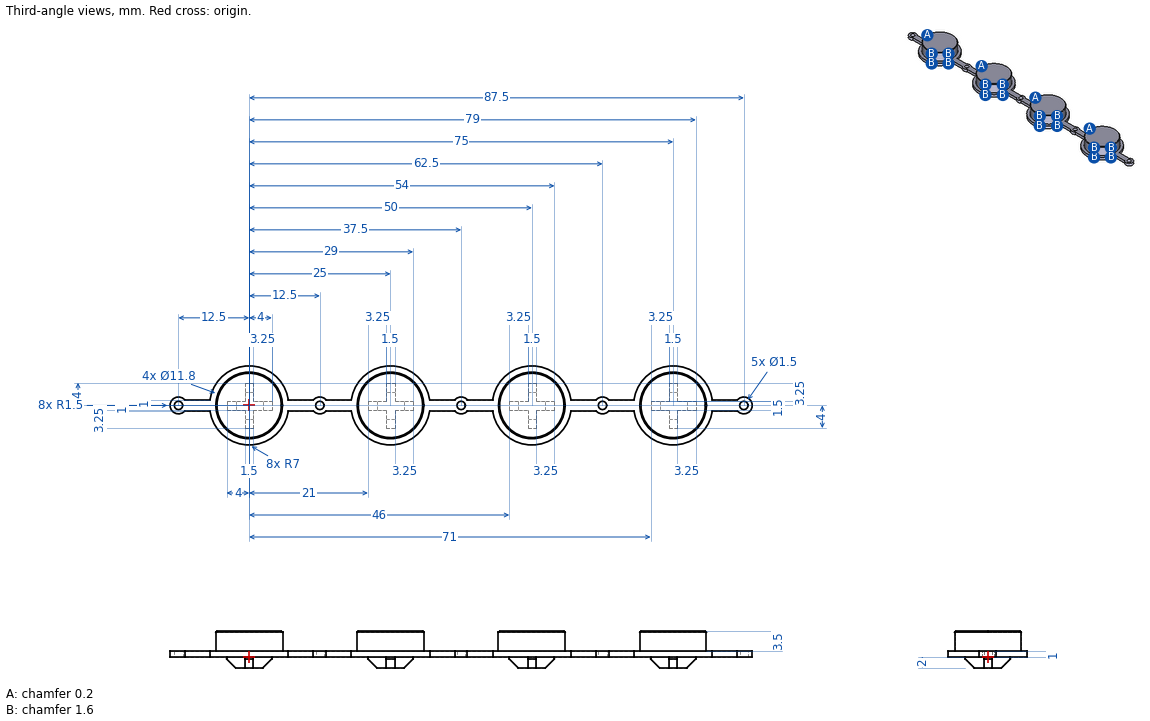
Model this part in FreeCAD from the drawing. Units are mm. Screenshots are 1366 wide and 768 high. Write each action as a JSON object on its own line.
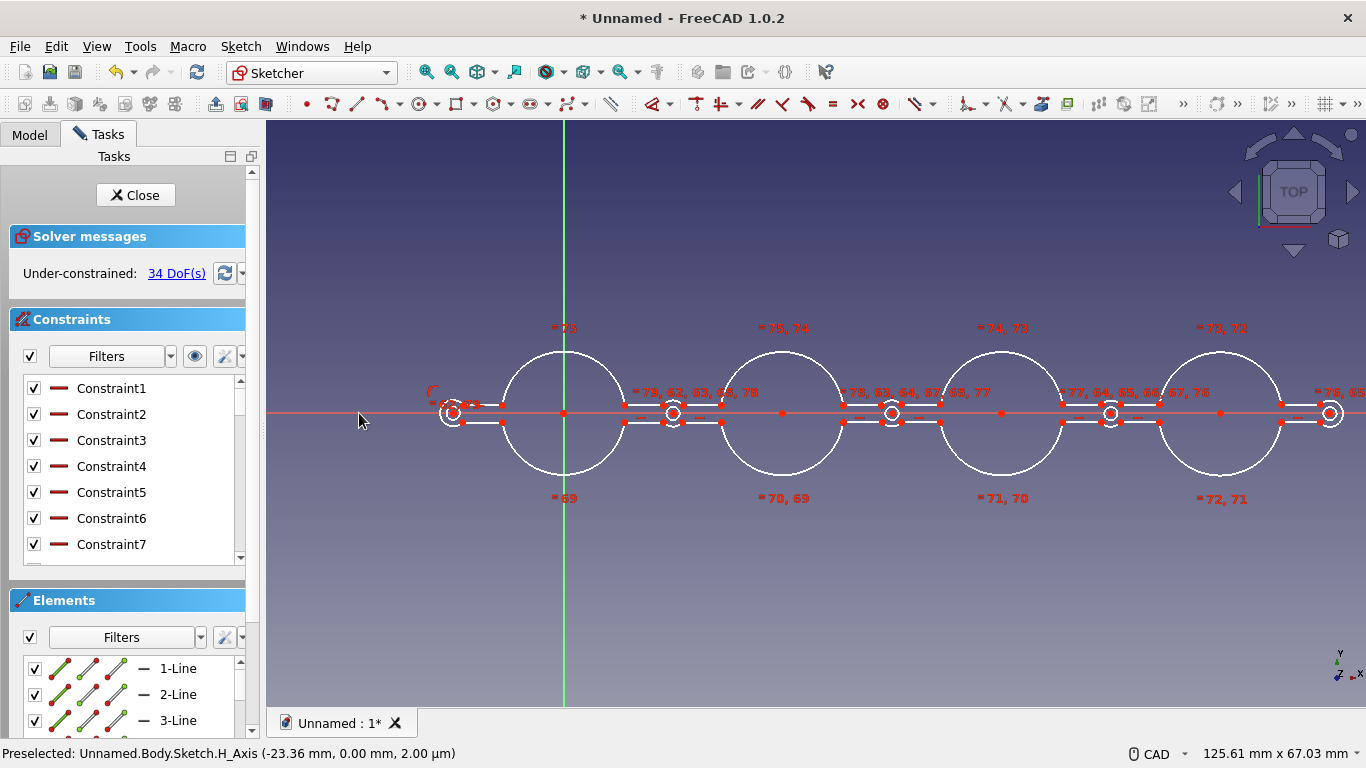
{"action": "left_click", "coordinate": [673, 414]}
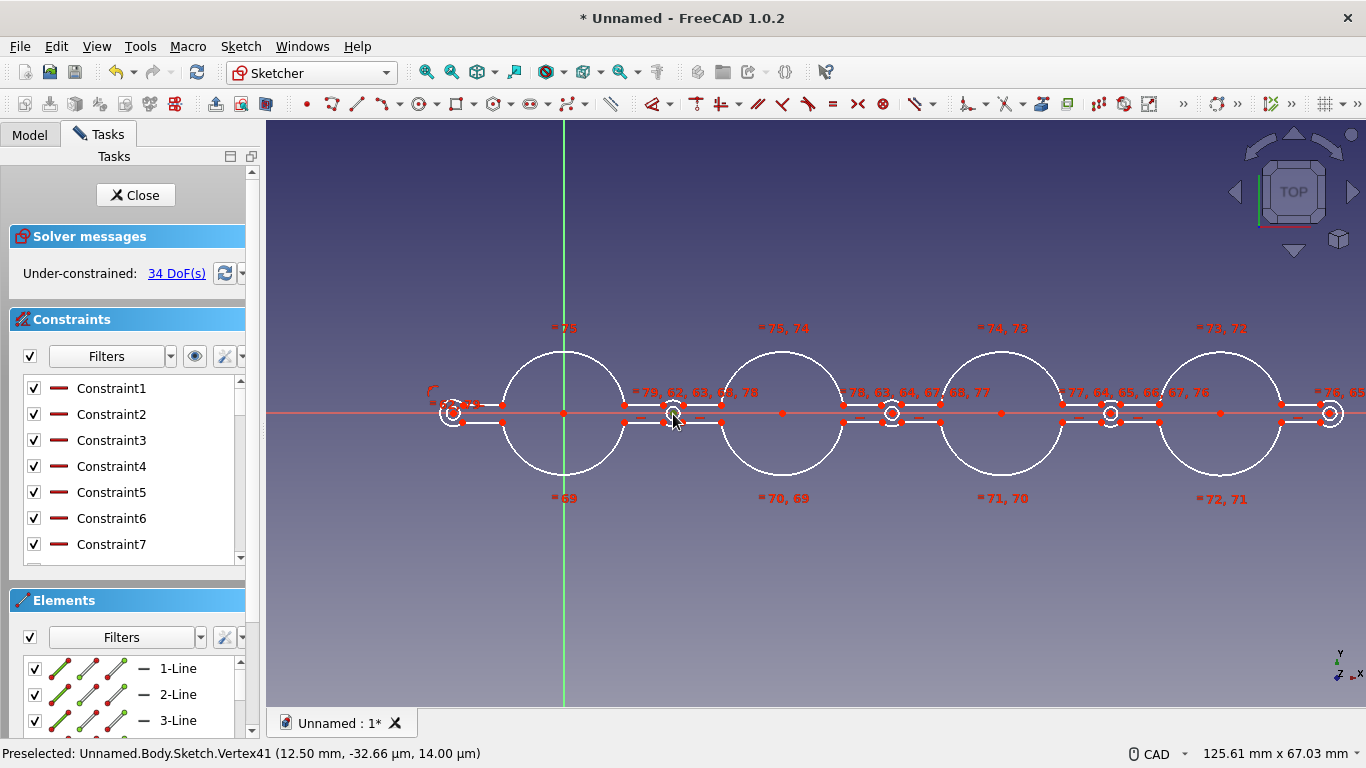
{"action": "left_click", "coordinate": [359, 413]}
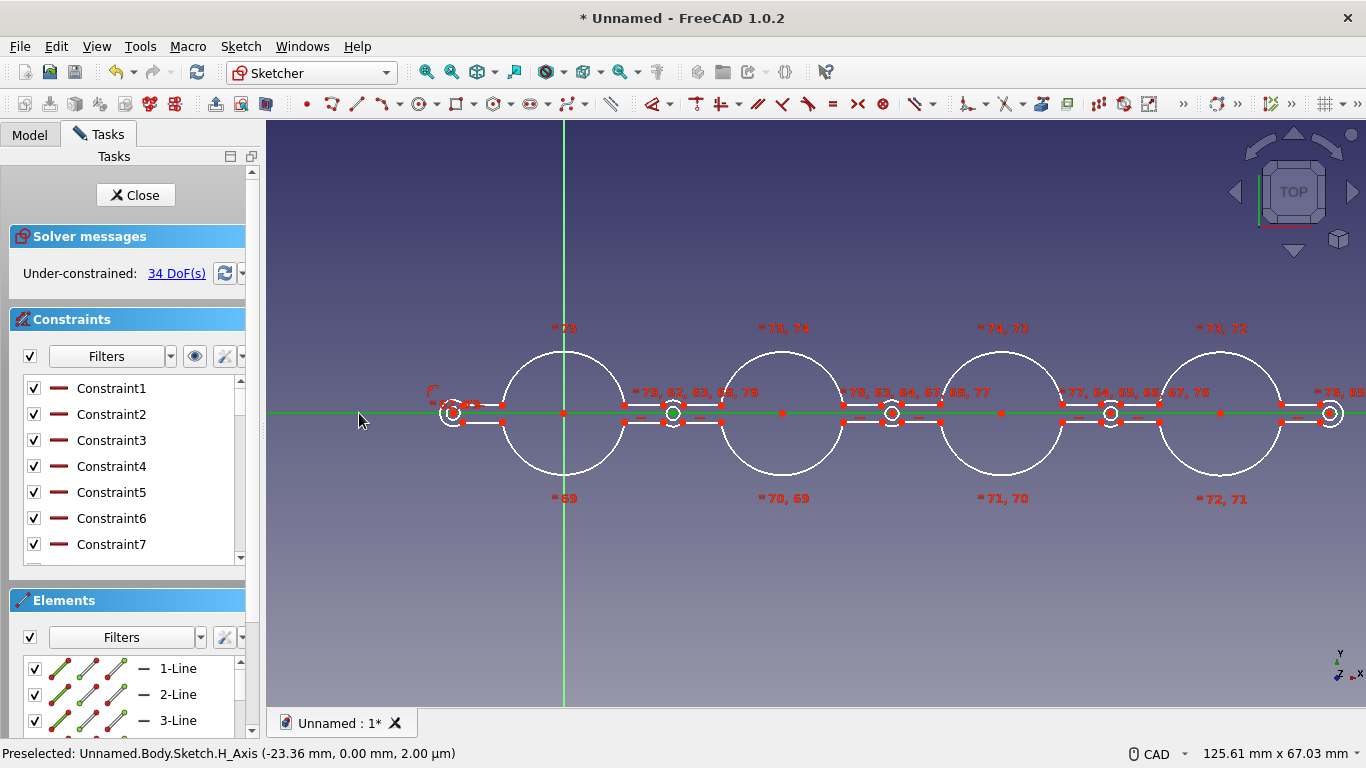
{"action": "key", "text": "c"}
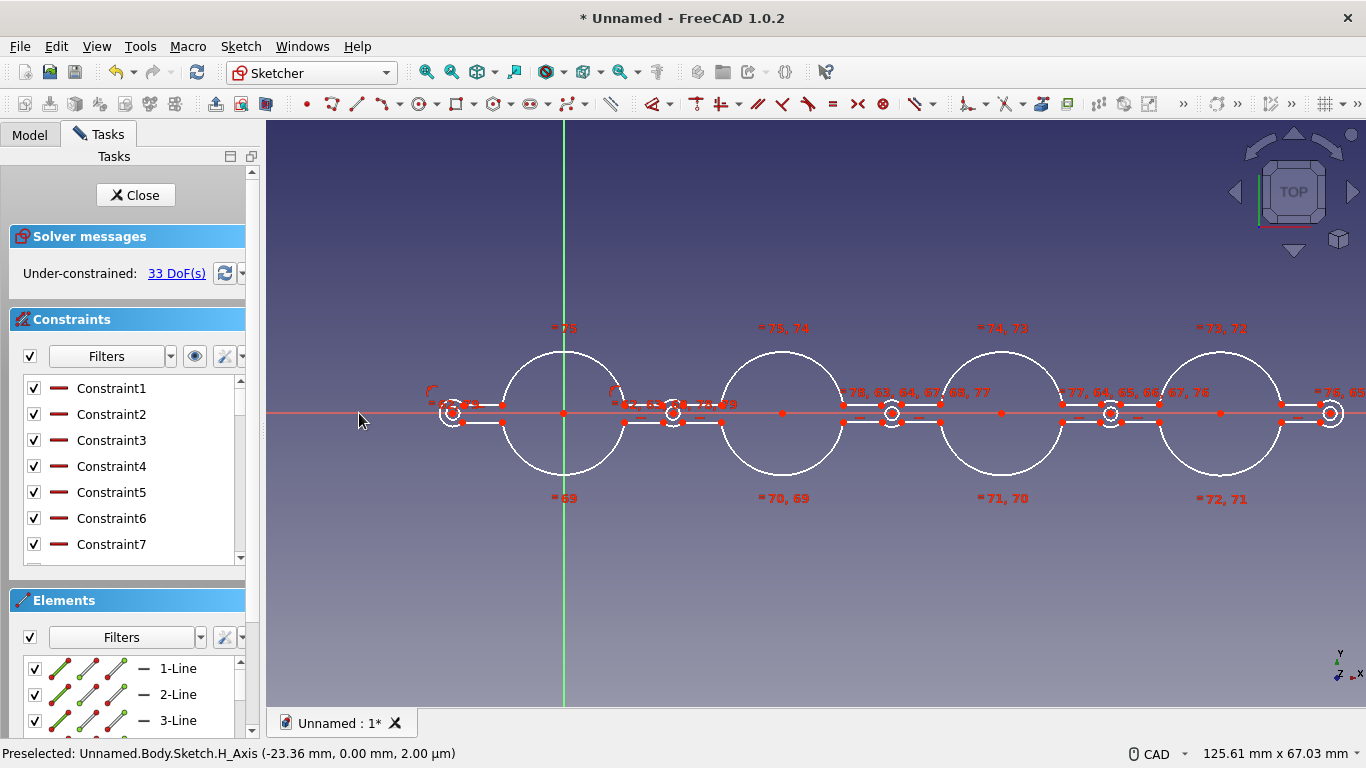
{"action": "left_click", "coordinate": [782, 414]}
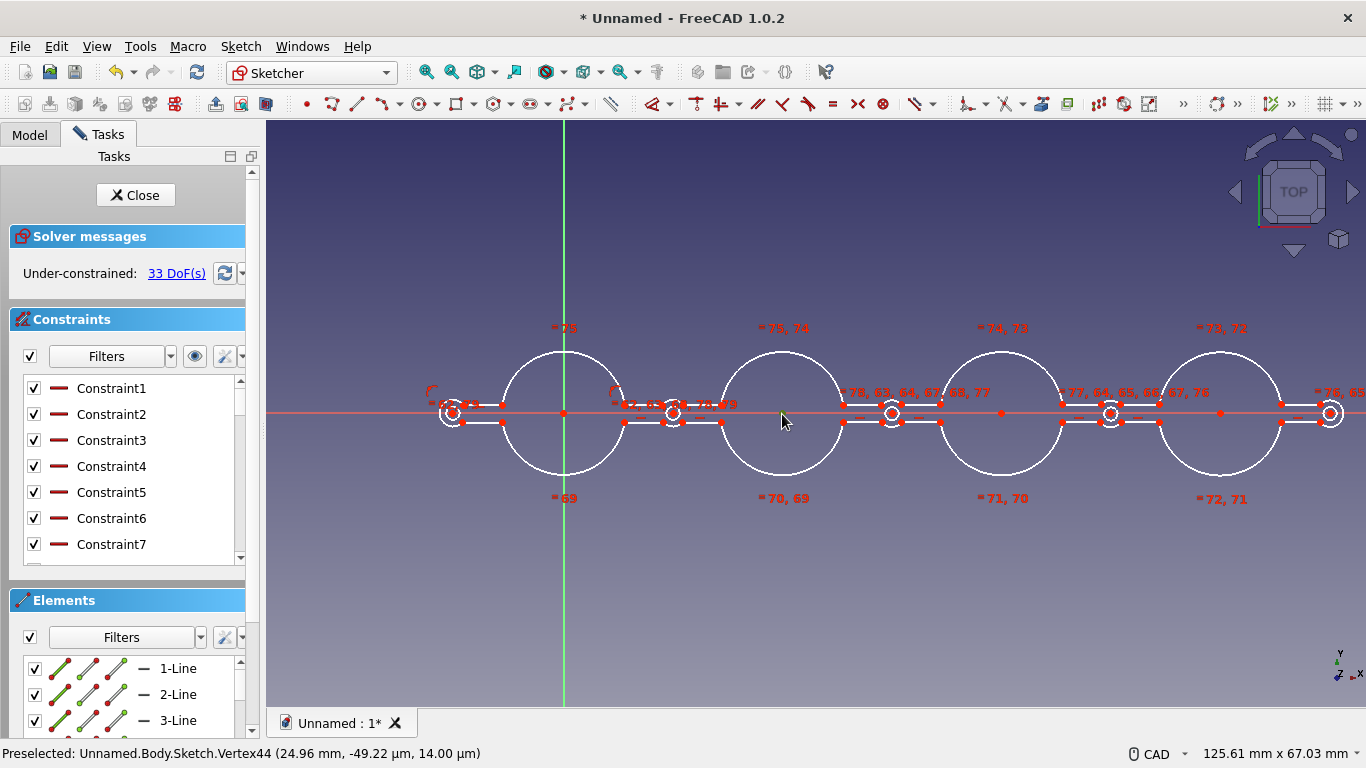
{"action": "left_click", "coordinate": [359, 413]}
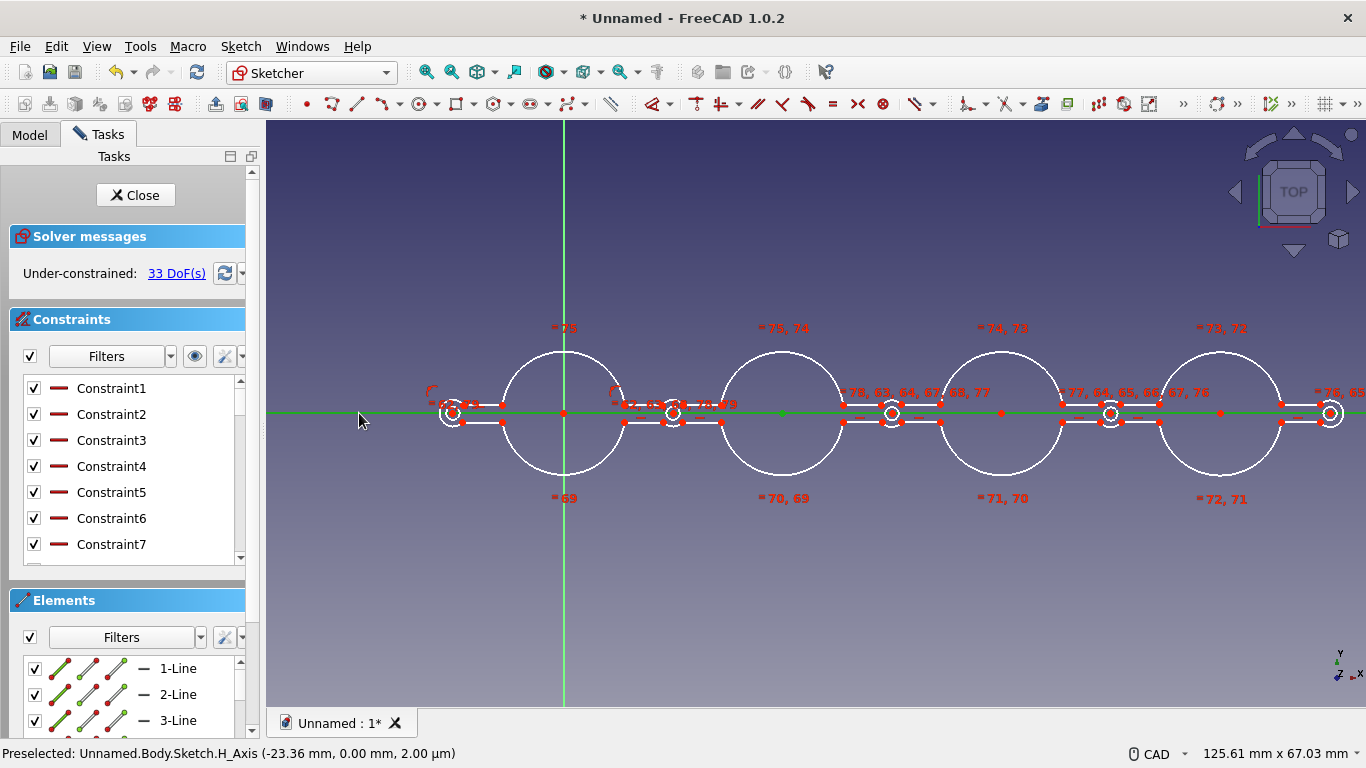
{"action": "key", "text": "c"}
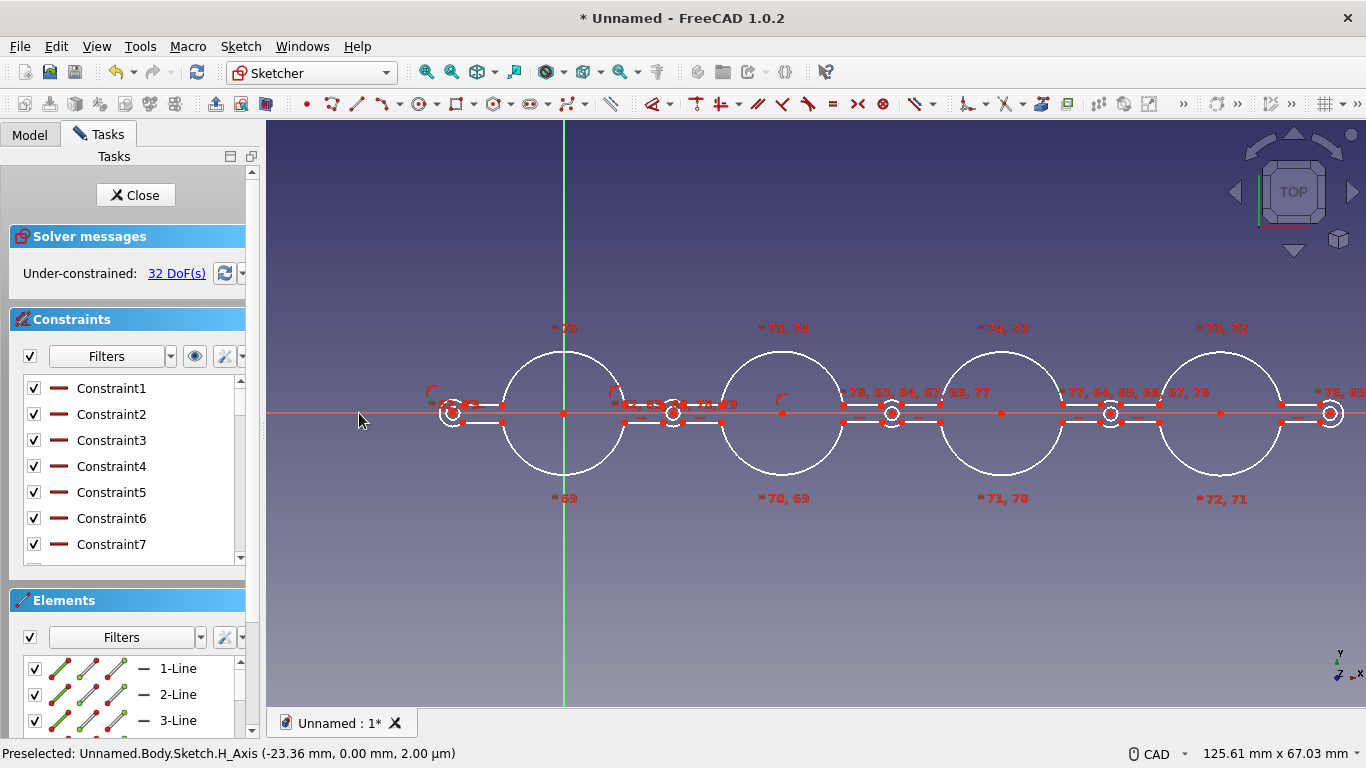
{"action": "left_click", "coordinate": [892, 414]}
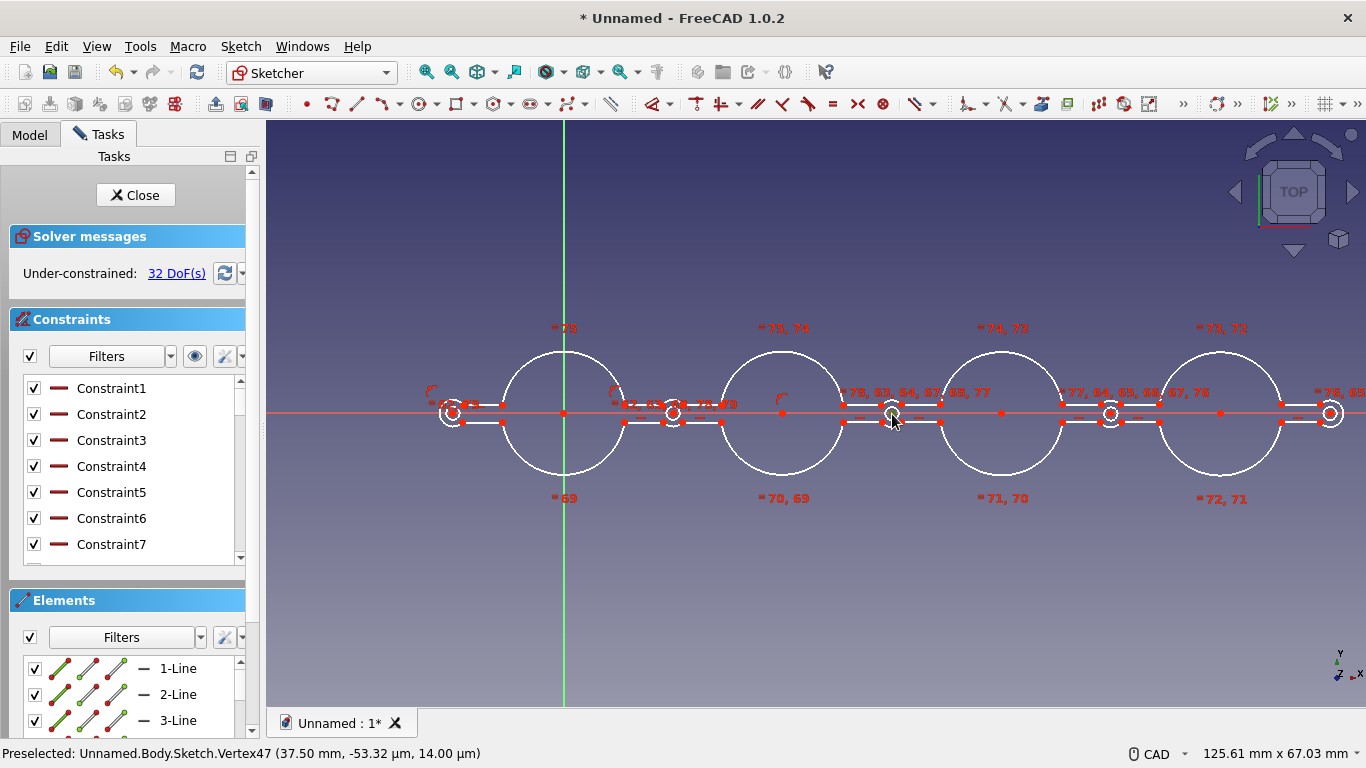
{"action": "left_click", "coordinate": [359, 413]}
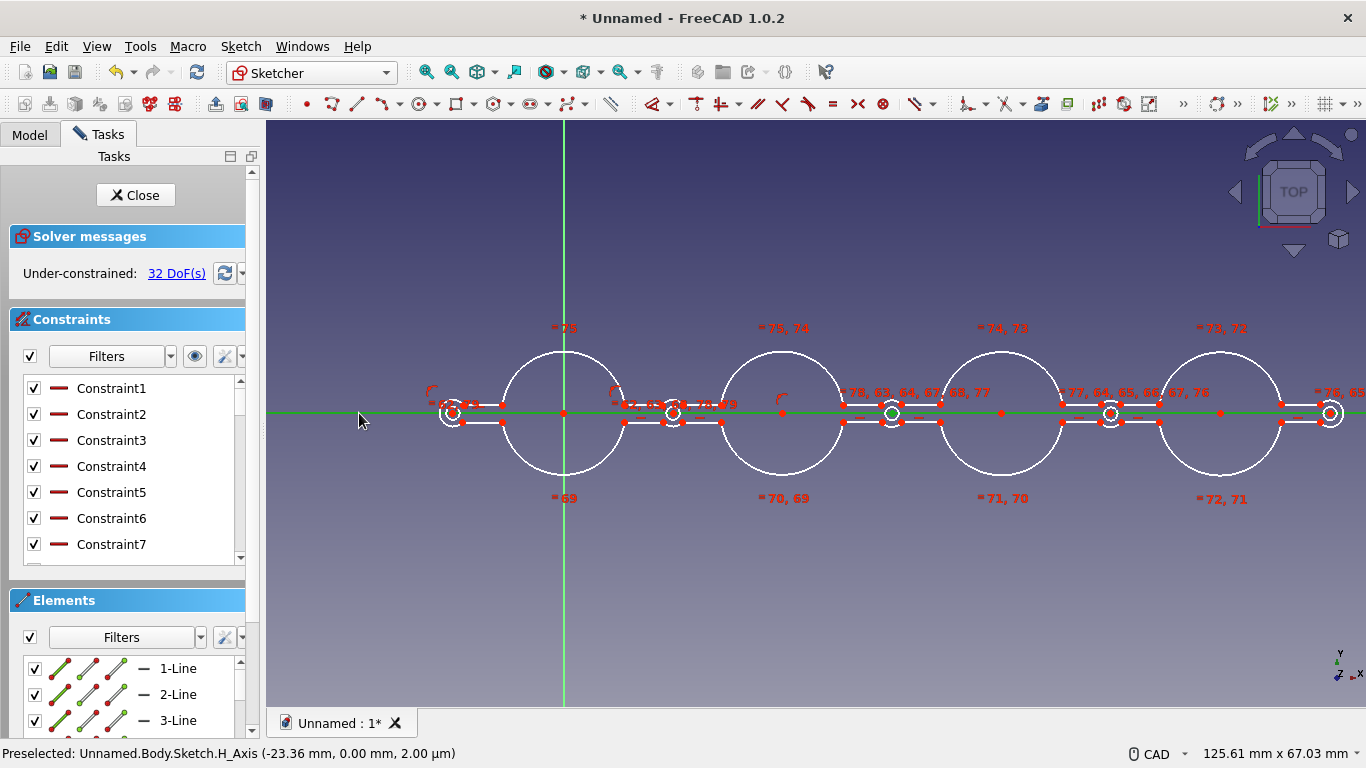
{"action": "key", "text": "c"}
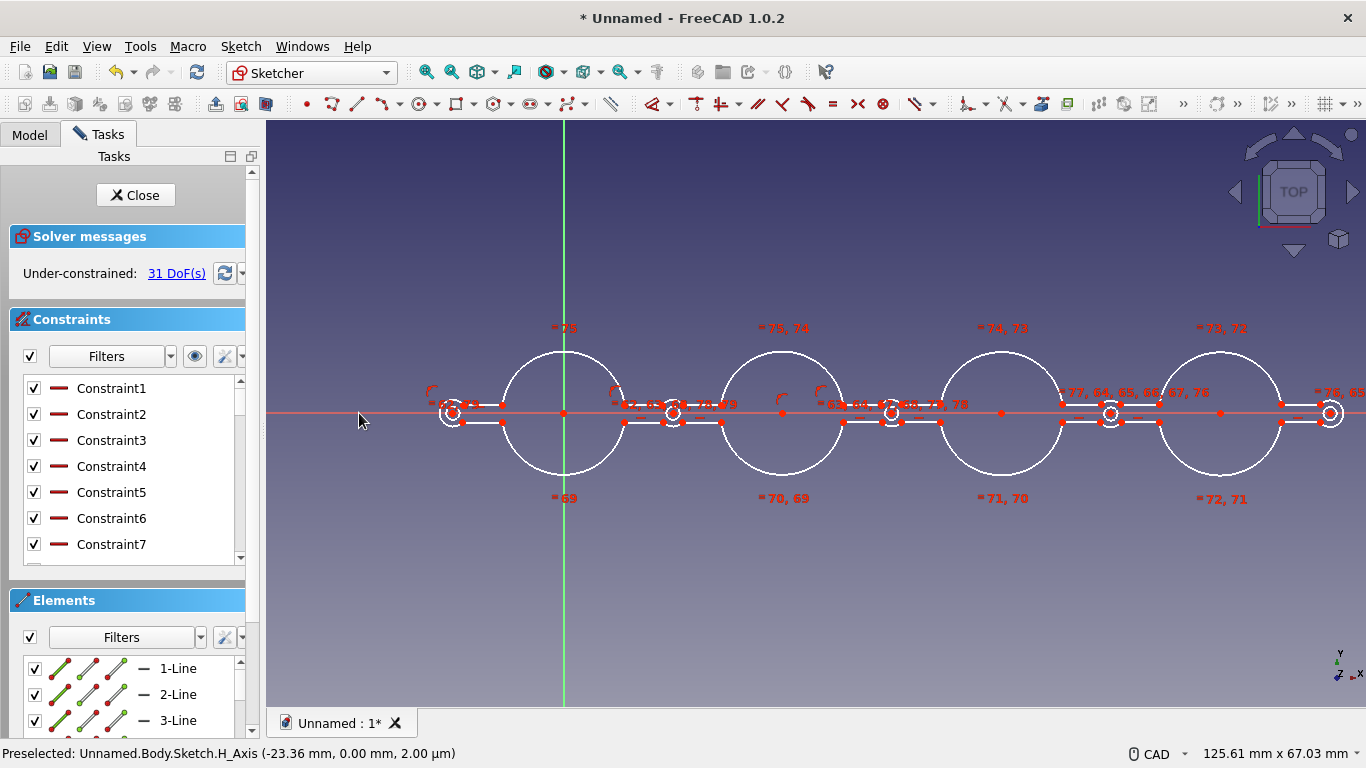
{"action": "left_click", "coordinate": [1002, 414]}